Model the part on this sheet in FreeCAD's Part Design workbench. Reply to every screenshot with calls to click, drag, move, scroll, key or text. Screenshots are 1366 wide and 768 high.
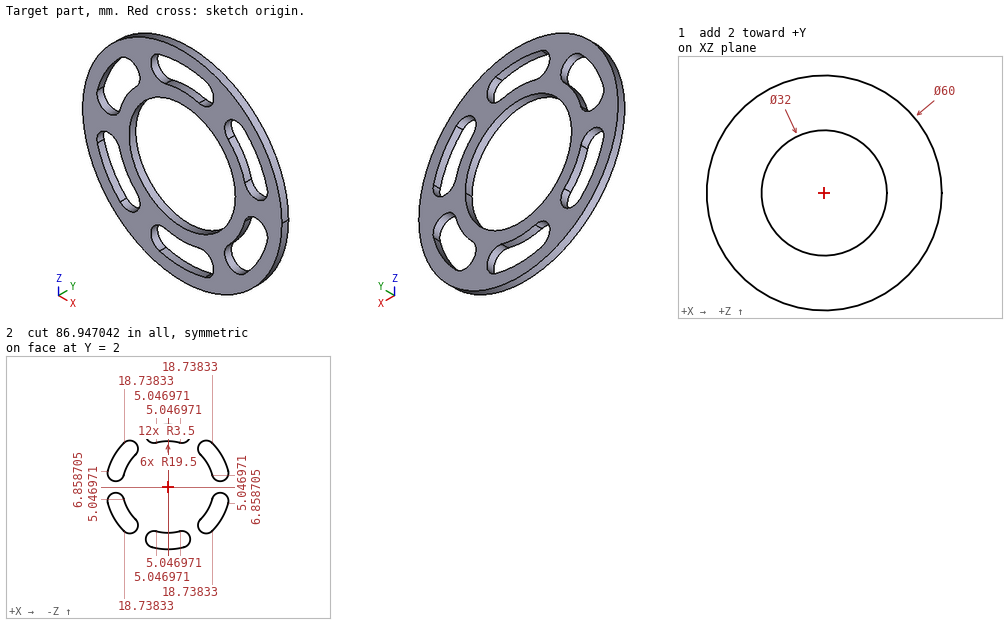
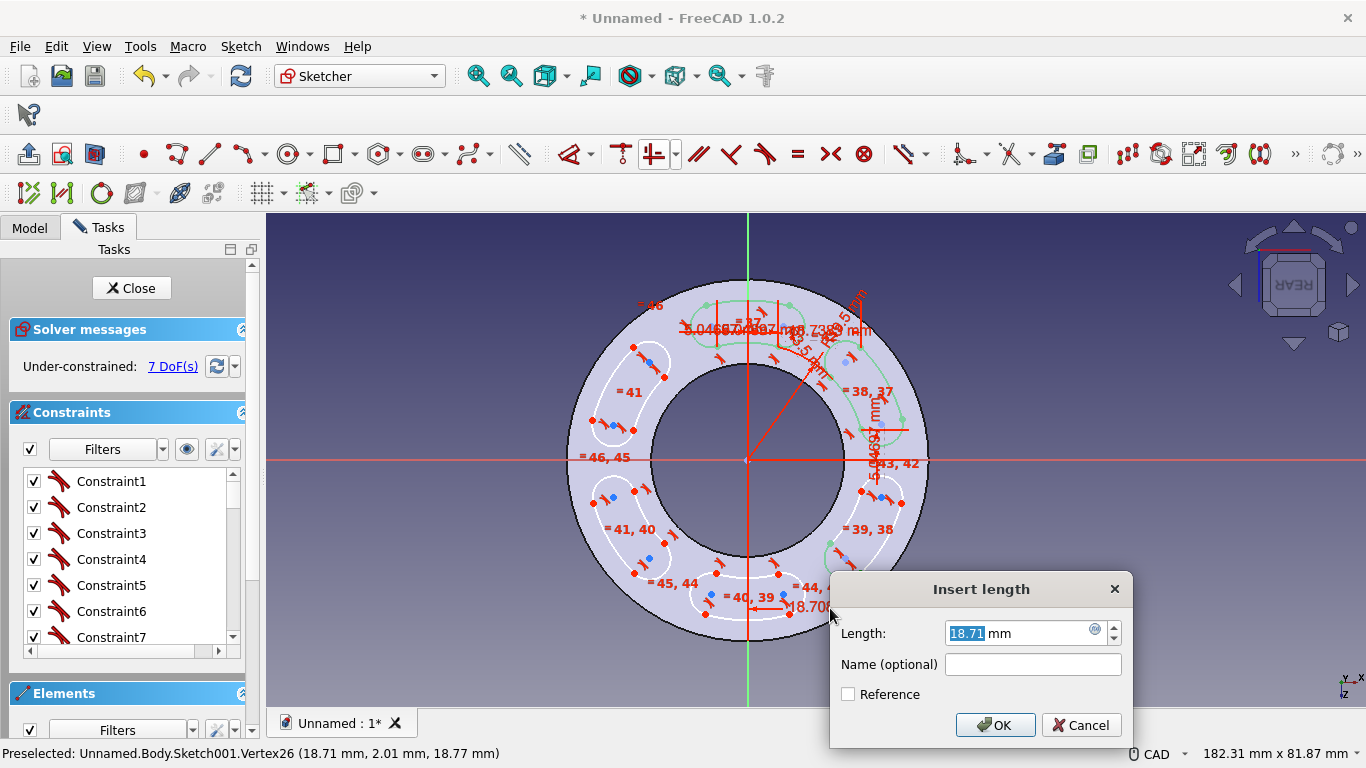
text(18.73833)
key(Return)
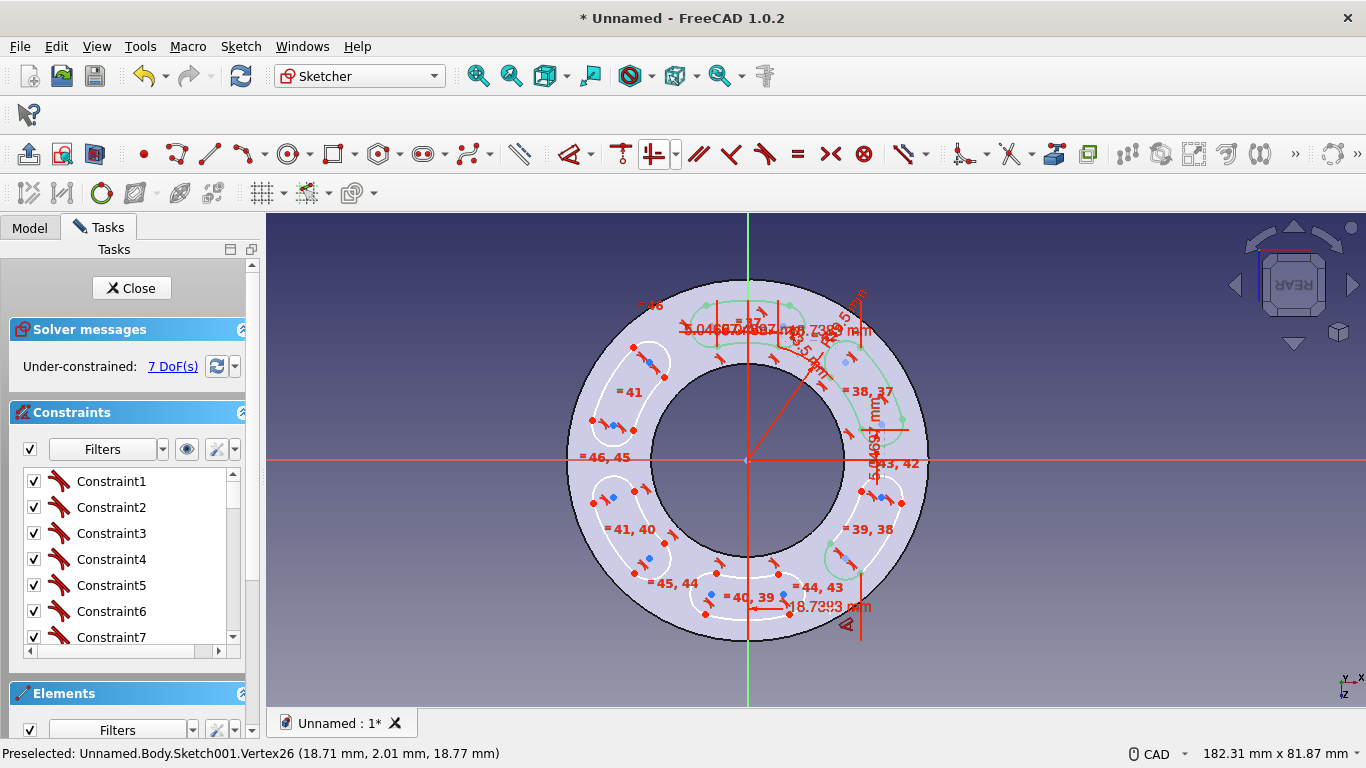
click(902, 503)
click(936, 482)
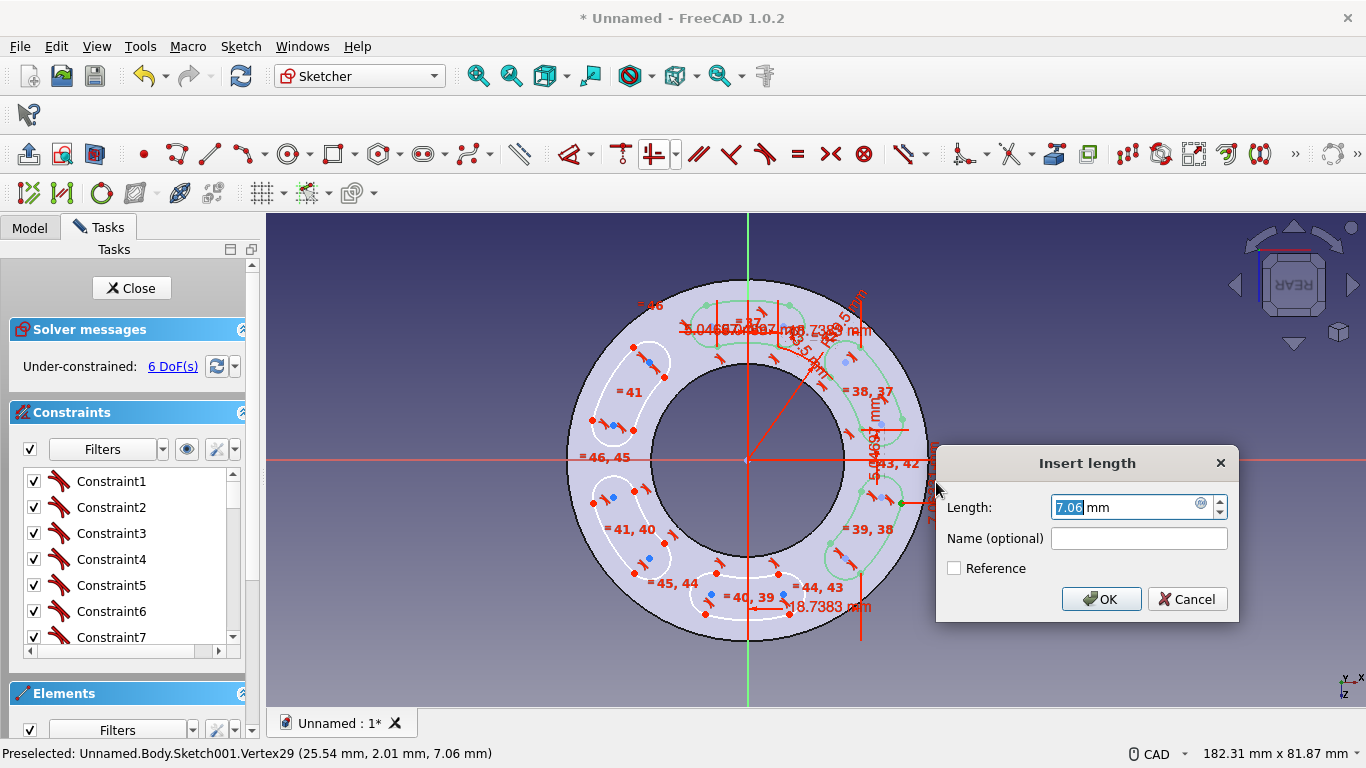
text(6.858705)
key(Return)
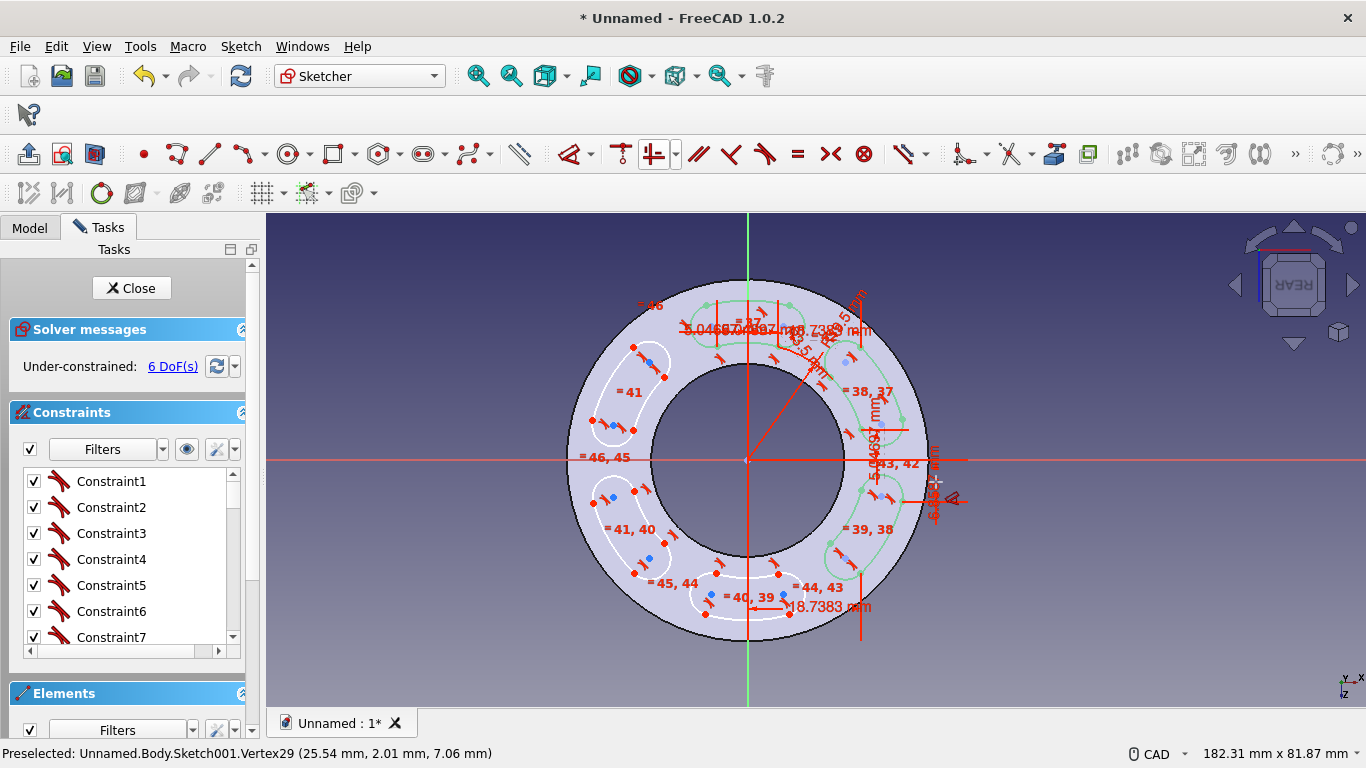
scroll(717, 574, up, 2)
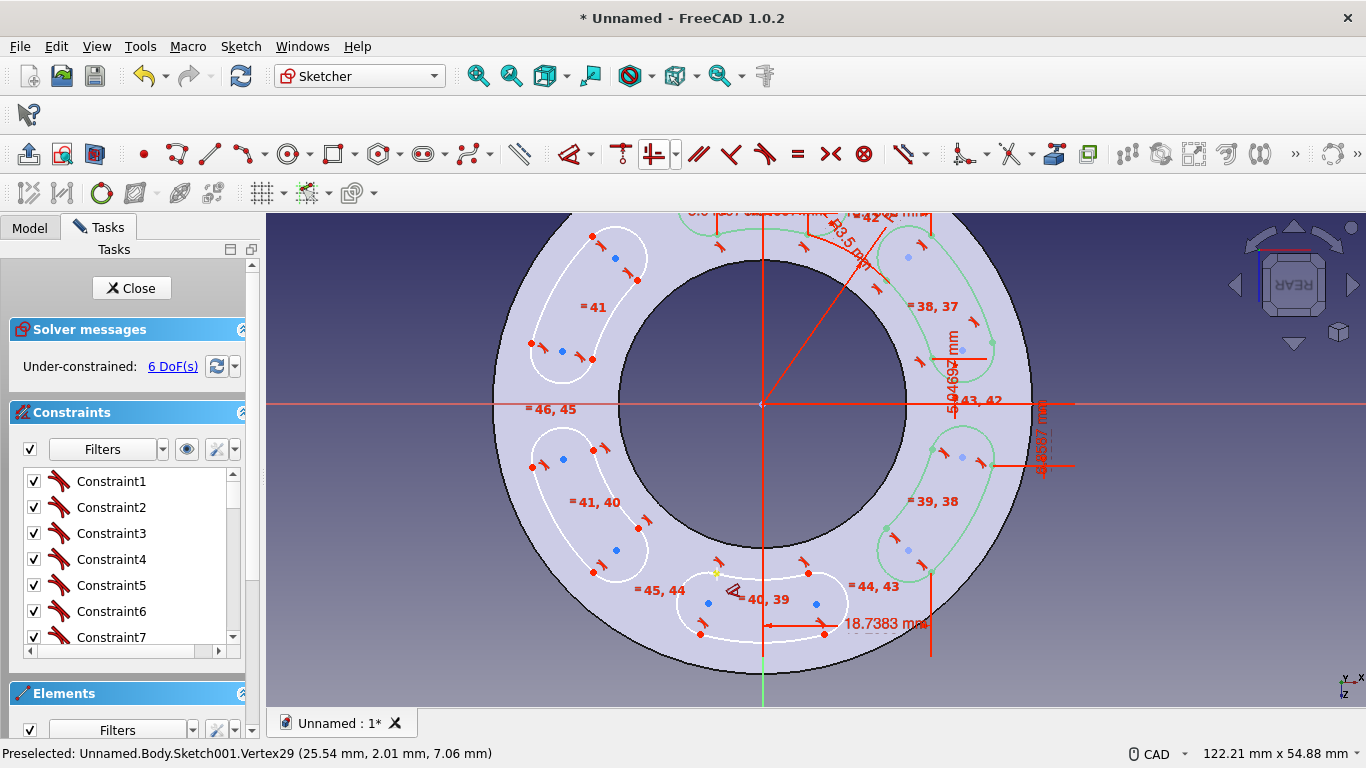
click(717, 574)
click(740, 608)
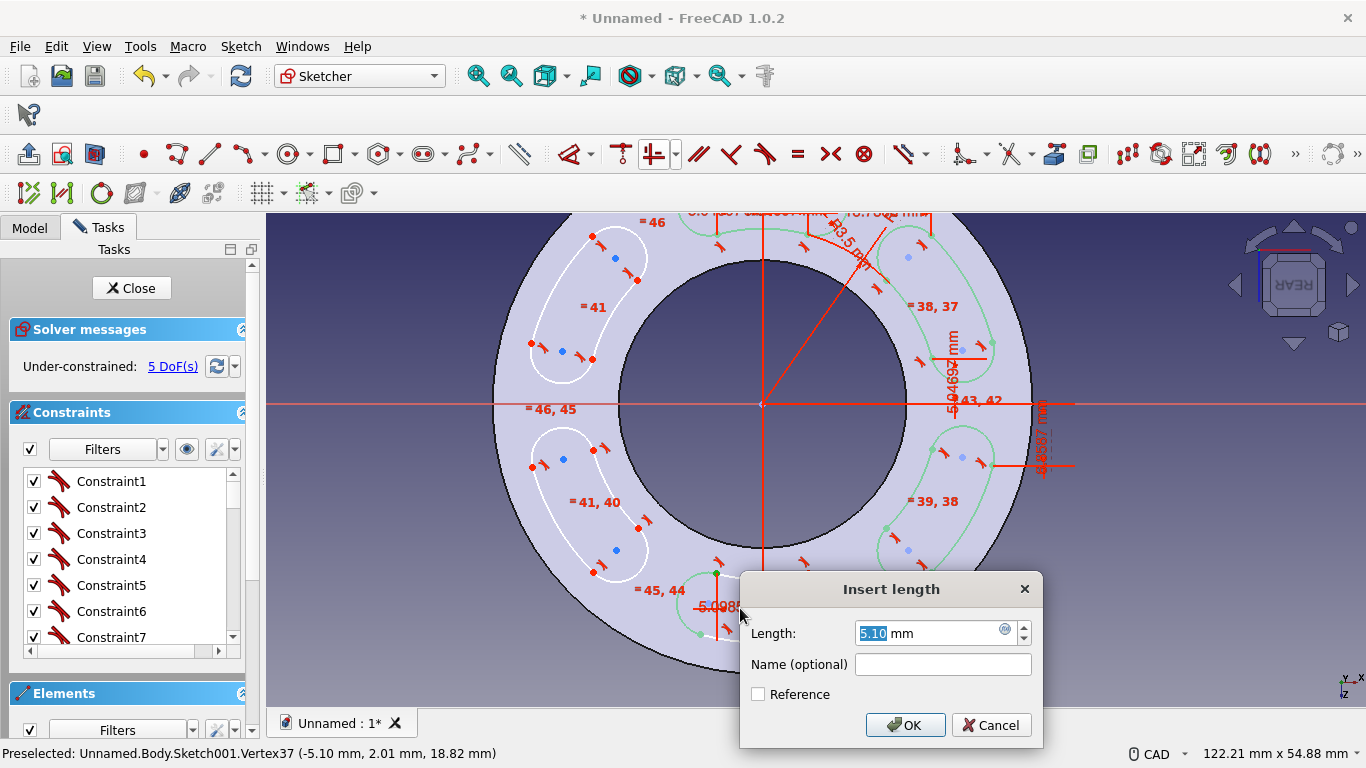
text(5.046971)
key(Return)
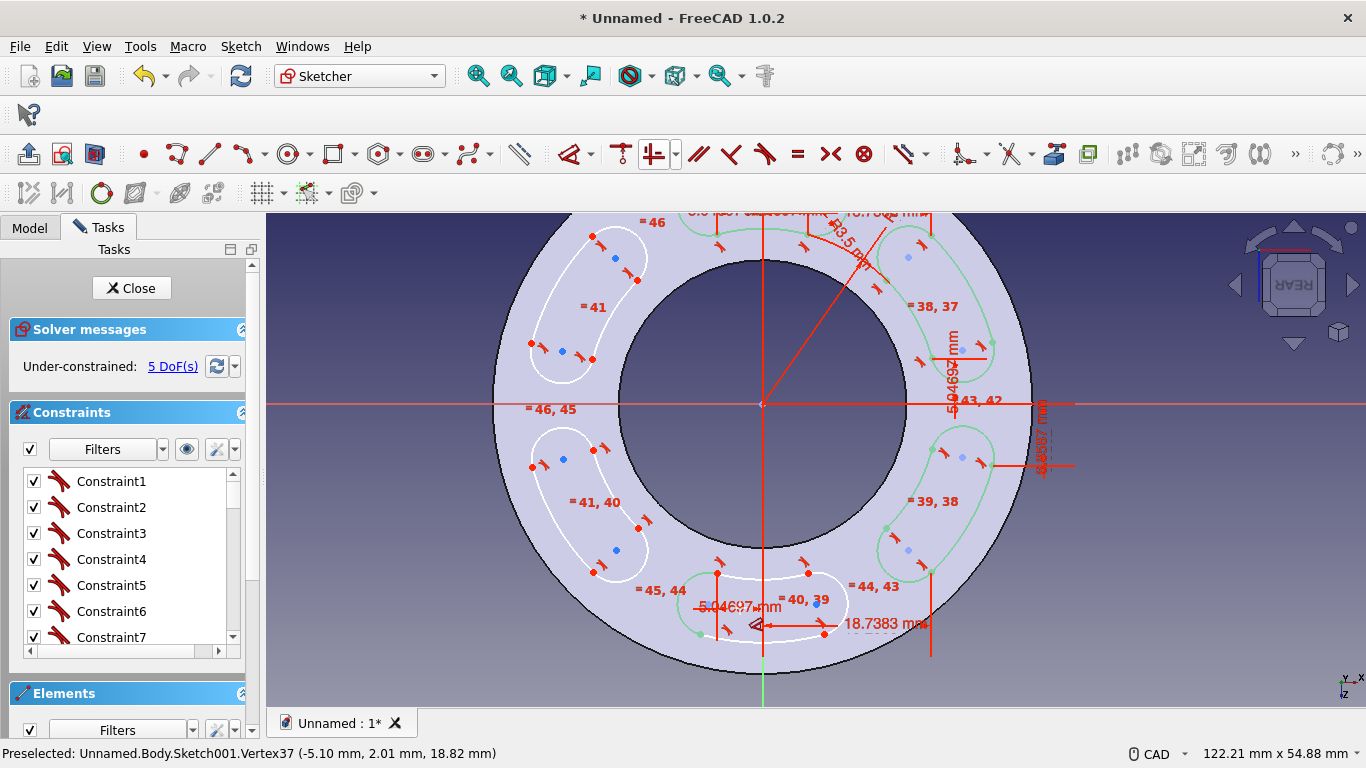
click(808, 574)
click(785, 370)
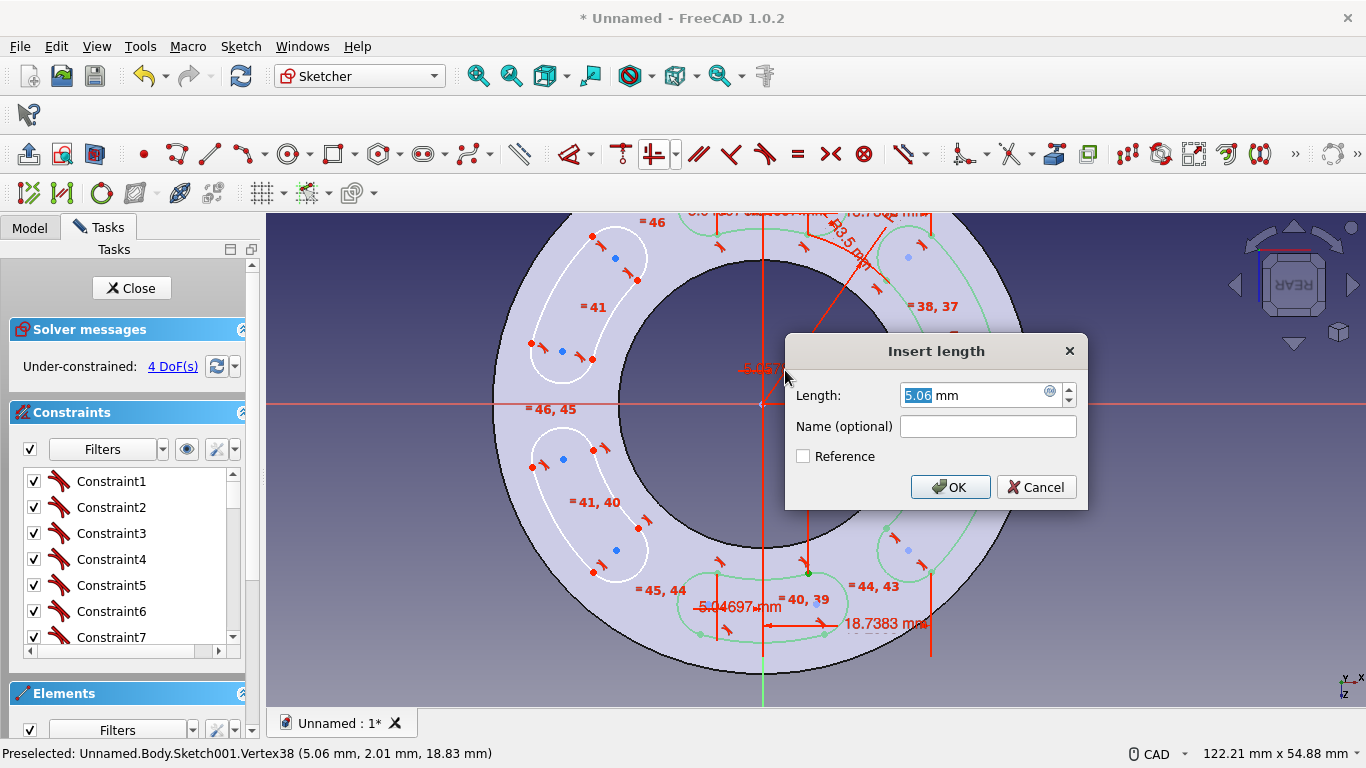
text(5.046971)
key(Return)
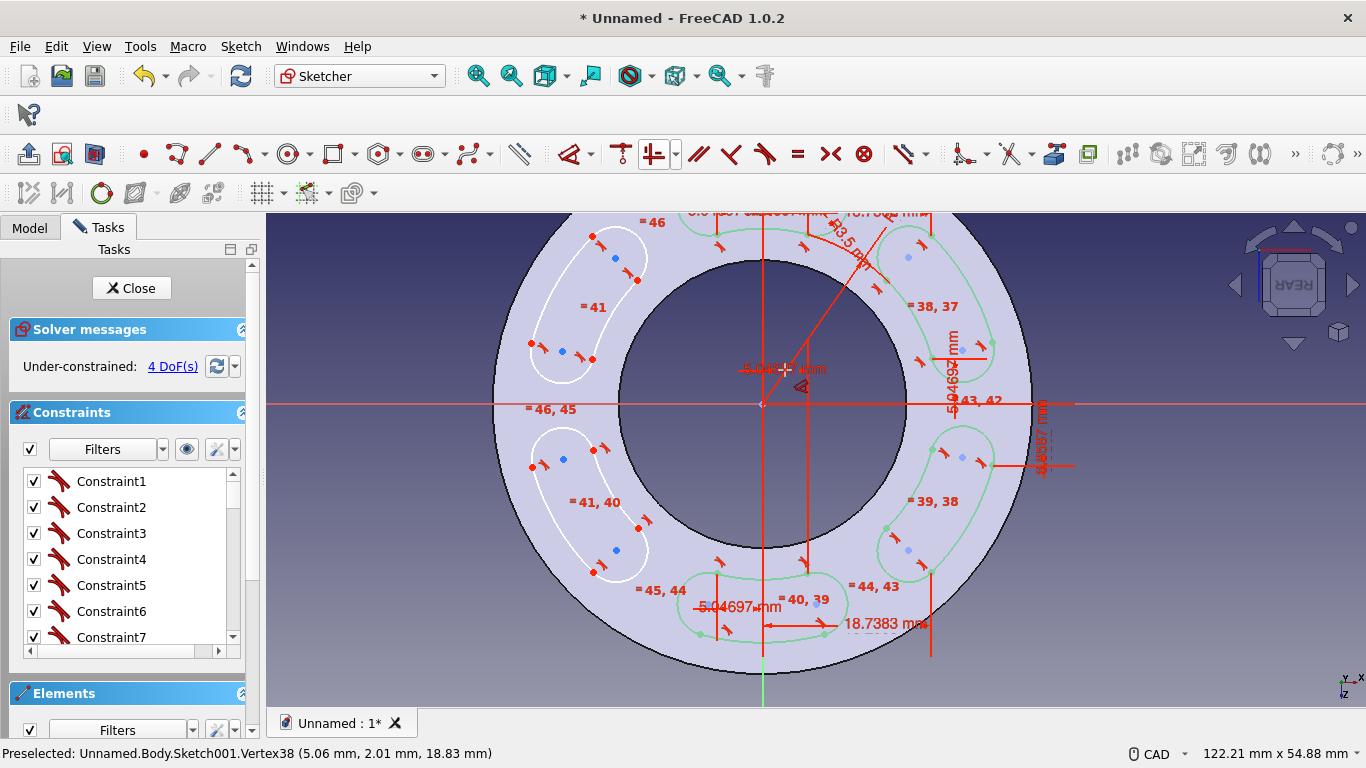
click(593, 451)
click(559, 444)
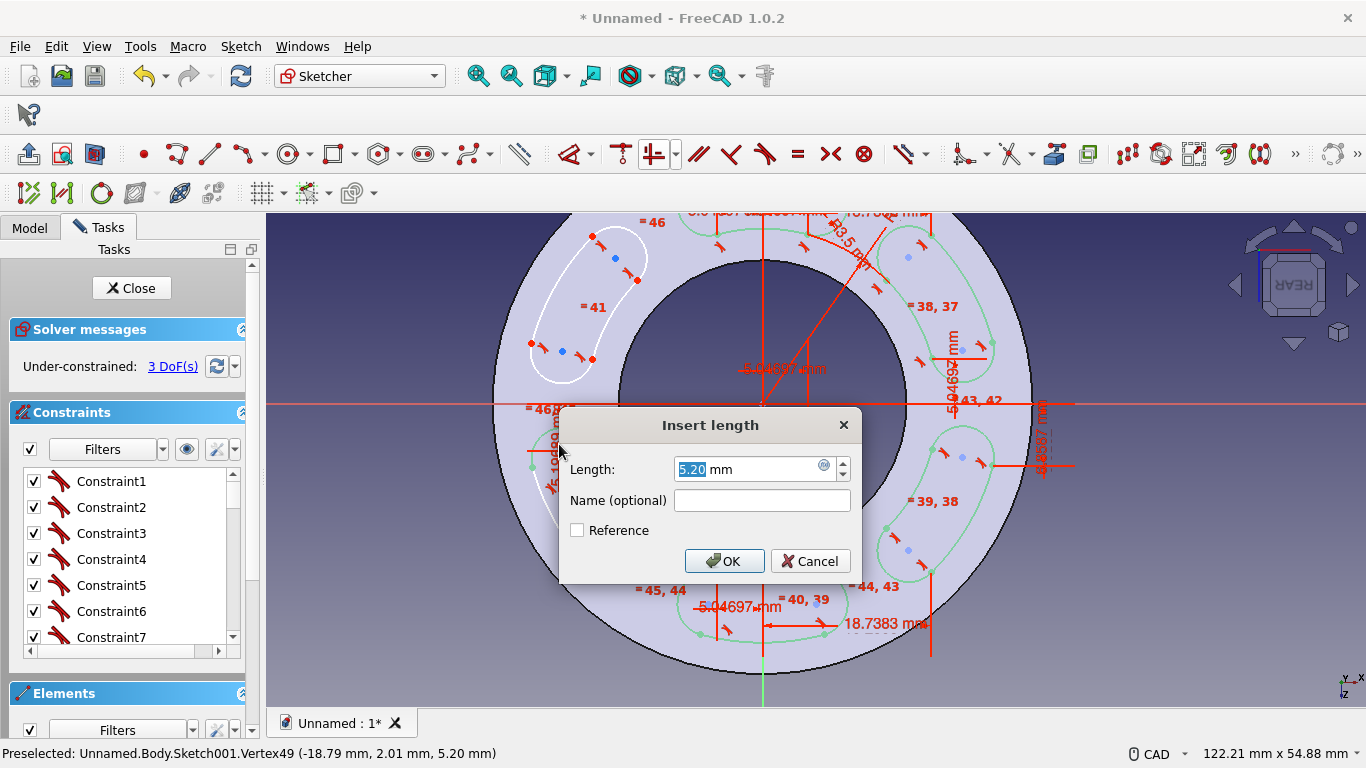
text(5.046971)
key(Return)